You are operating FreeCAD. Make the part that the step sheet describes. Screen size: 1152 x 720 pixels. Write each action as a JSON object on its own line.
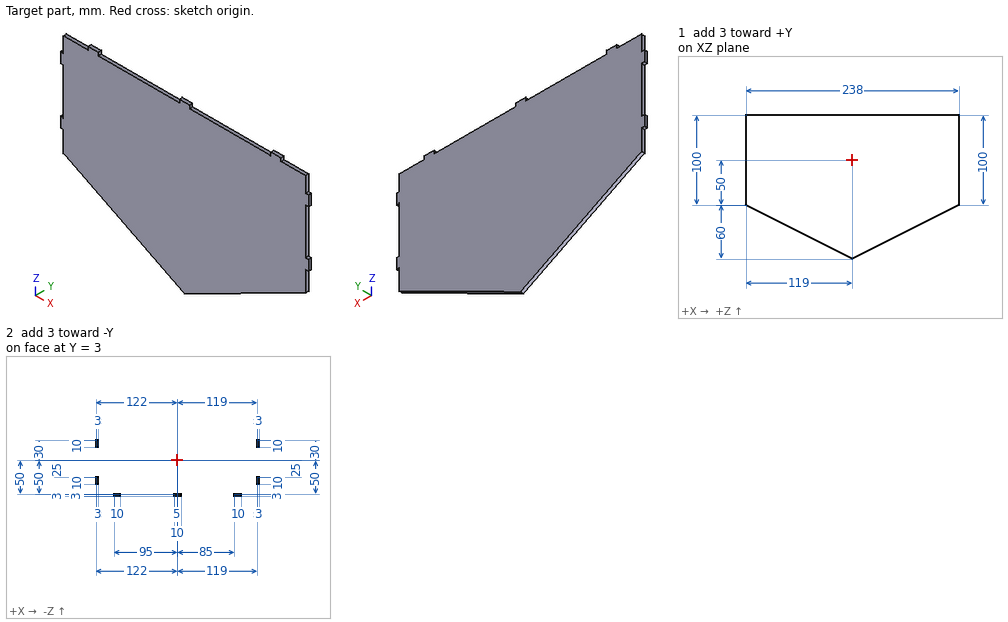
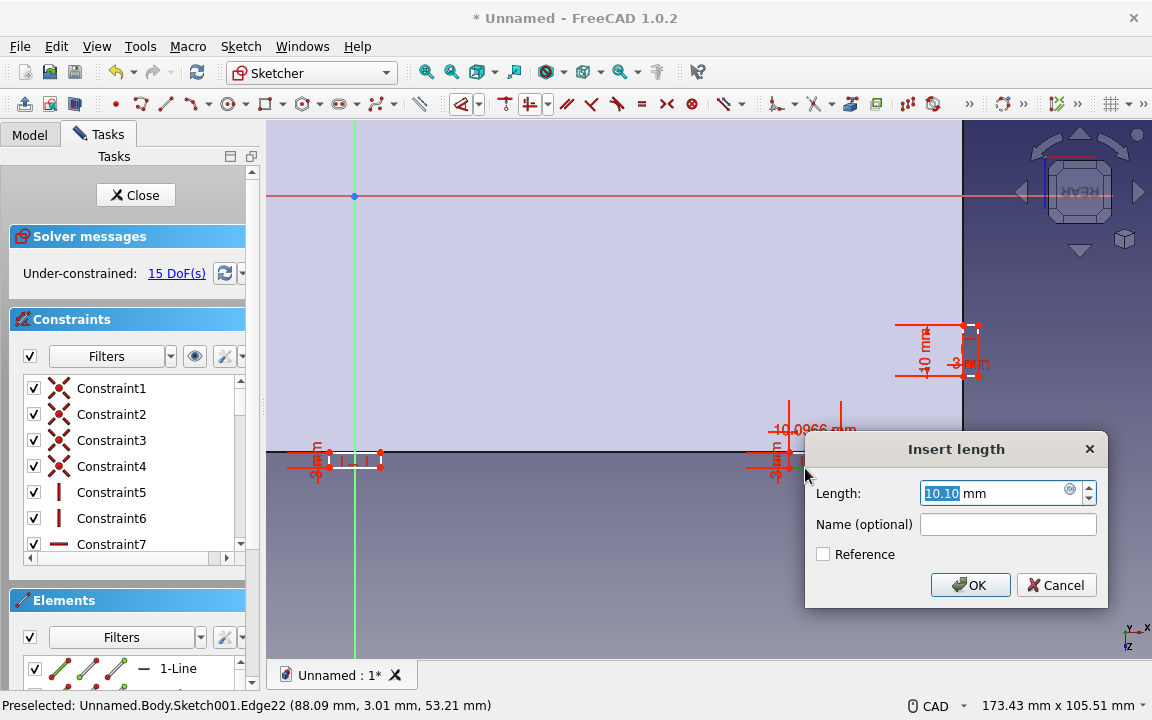
{"action": "type", "text": "10"}
{"action": "key", "text": "Return"}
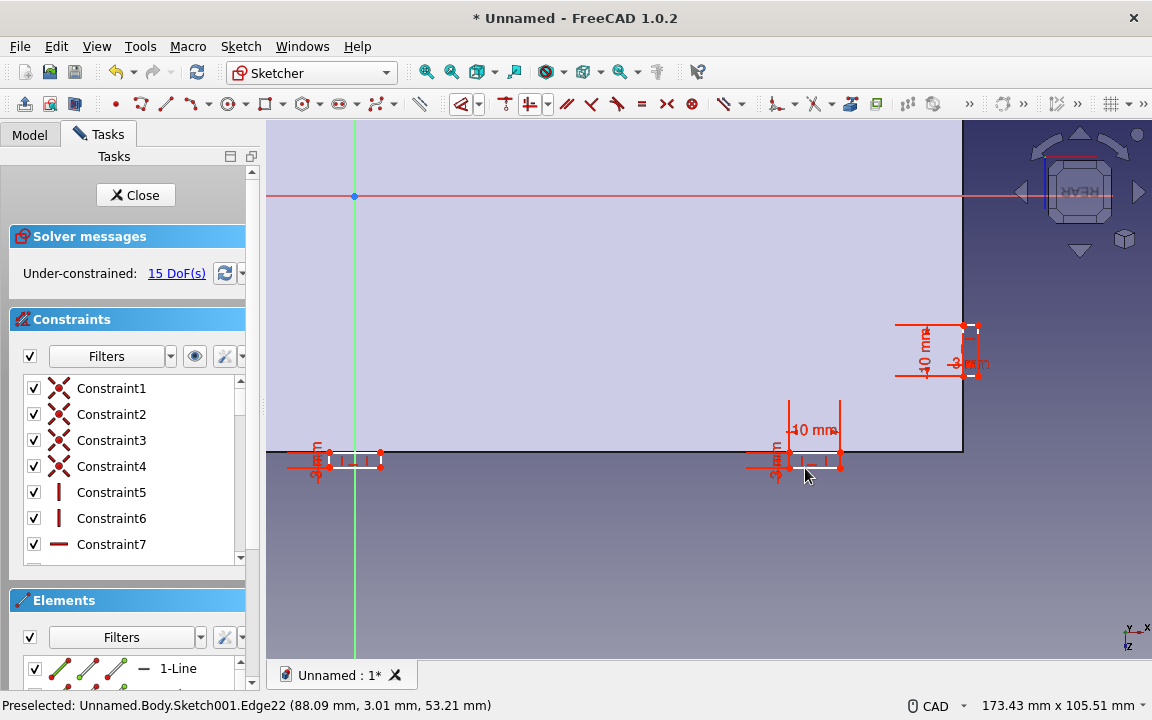
{"action": "scroll", "coordinate": [345, 468], "scroll_direction": "up", "scroll_amount": 2}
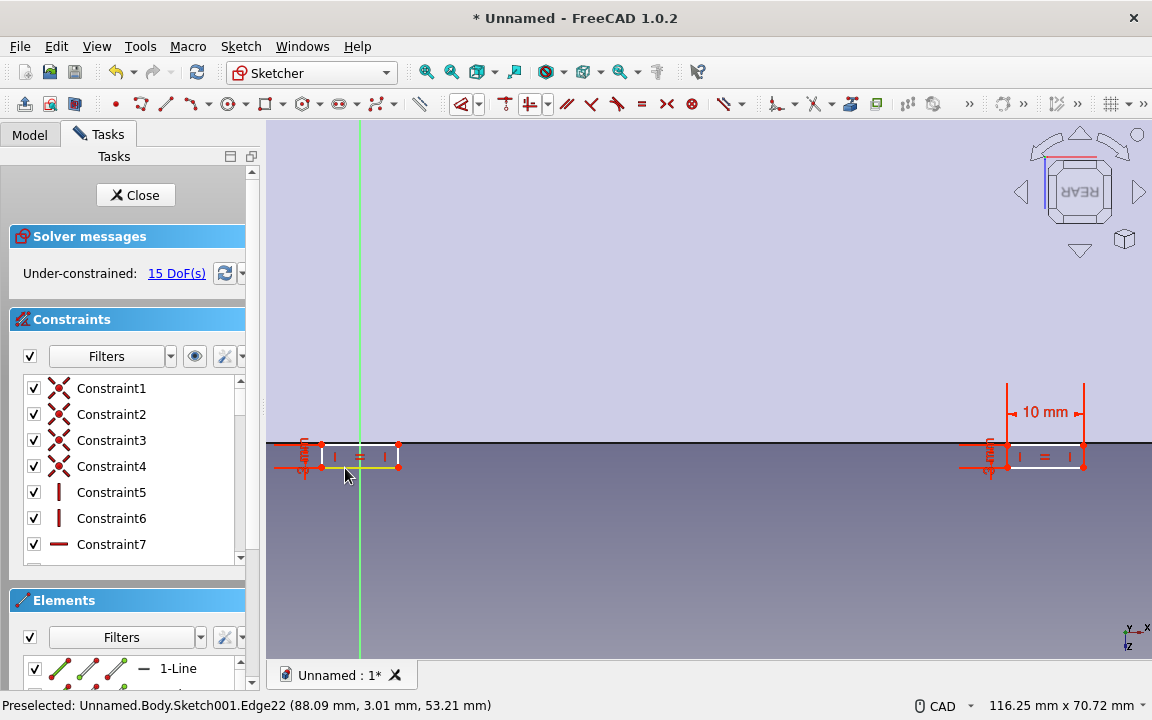
{"action": "left_click", "coordinate": [345, 468]}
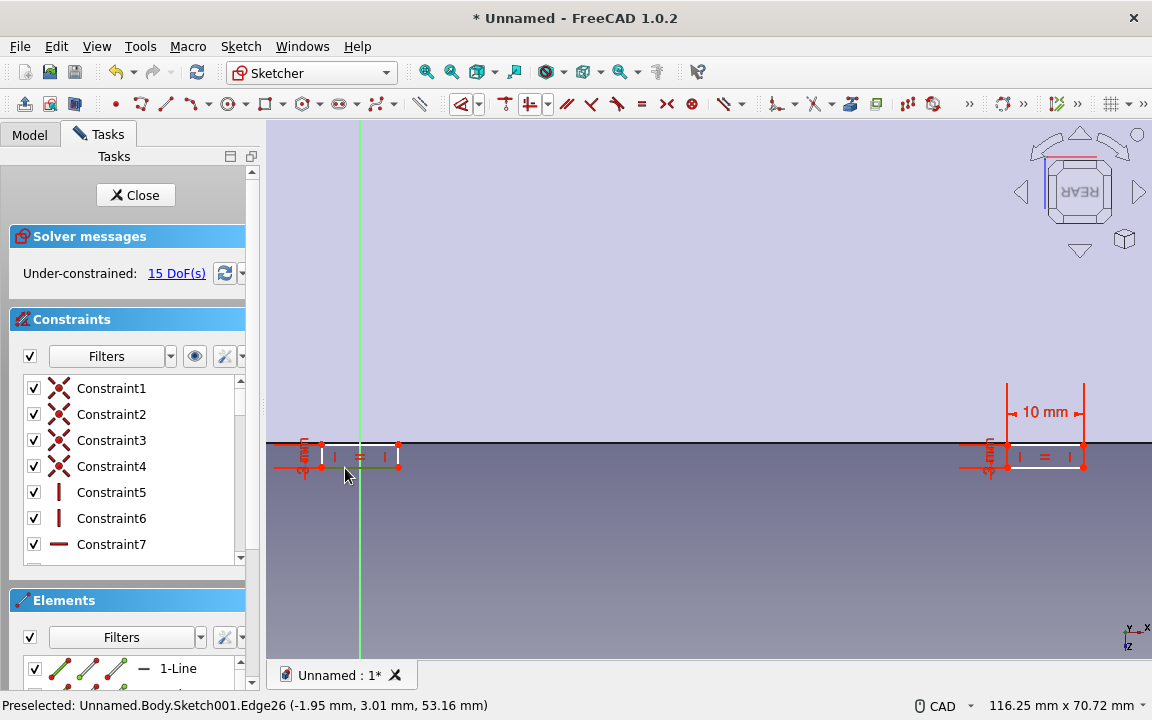
{"action": "key", "text": "l"}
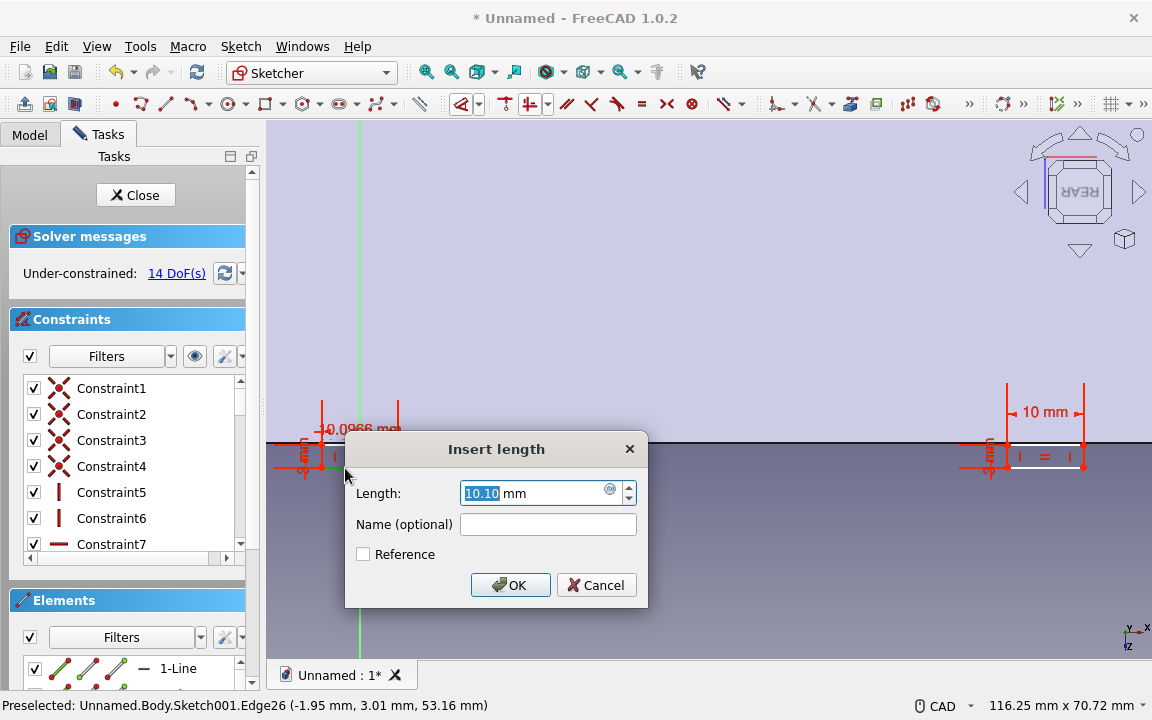
{"action": "type", "text": "10"}
{"action": "key", "text": "Return"}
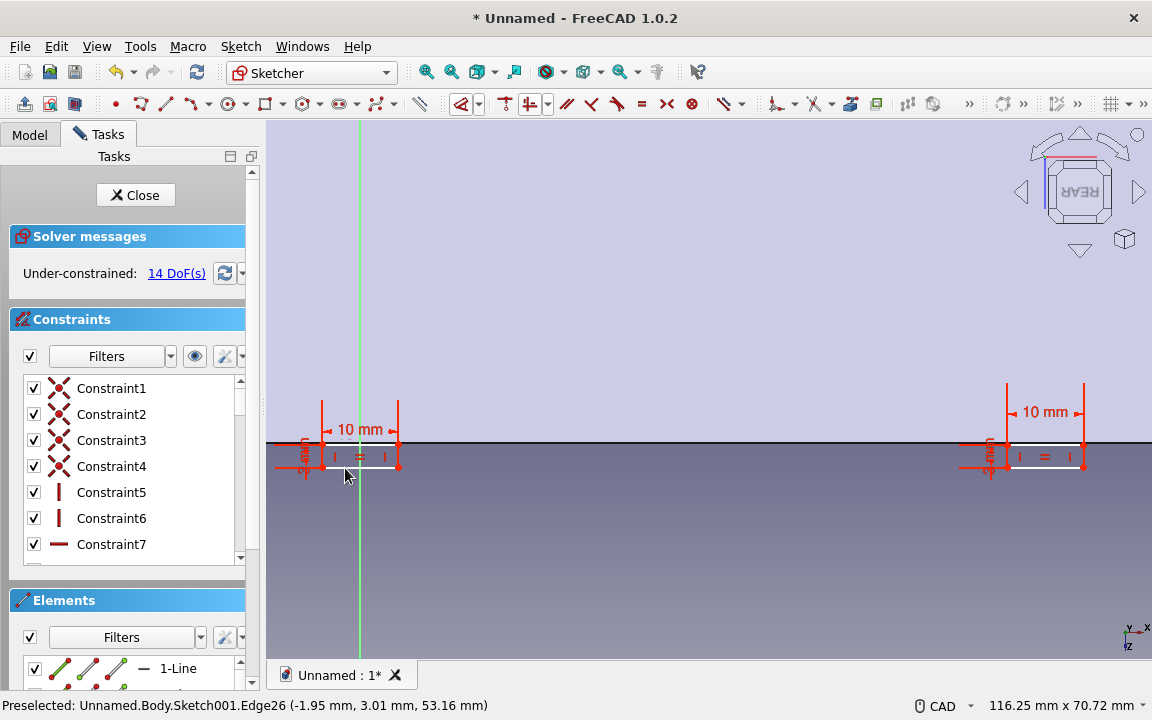
{"action": "left_click", "coordinate": [322, 445]}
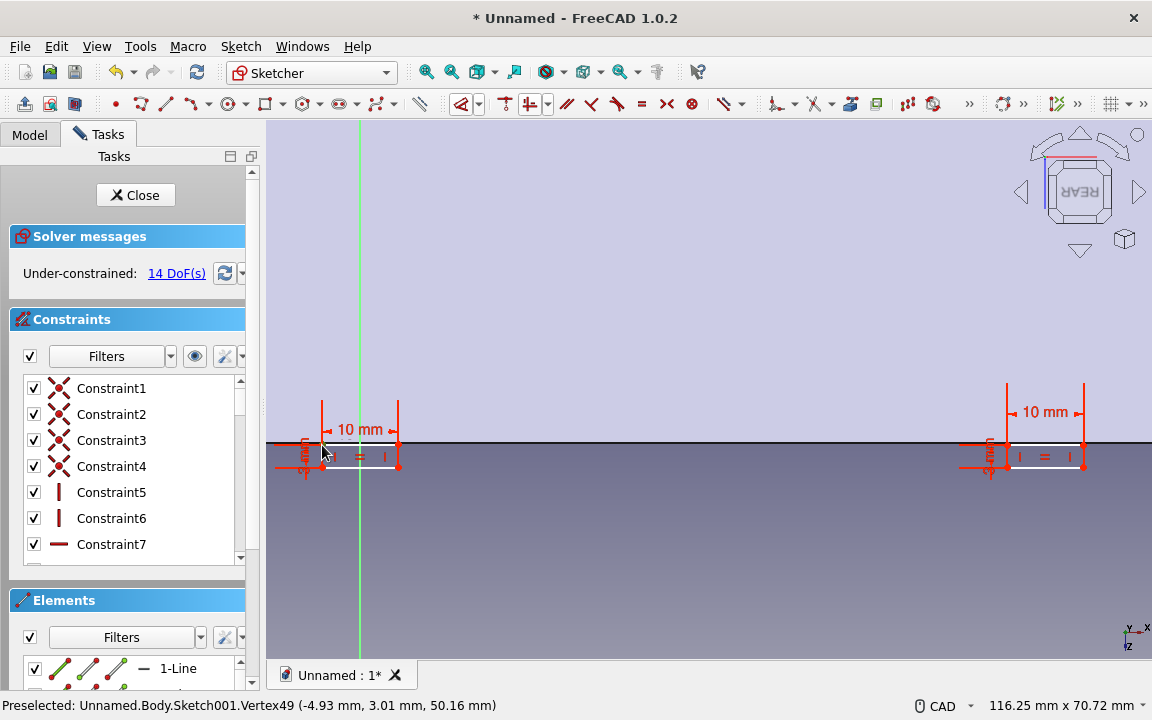
{"action": "key", "text": "l"}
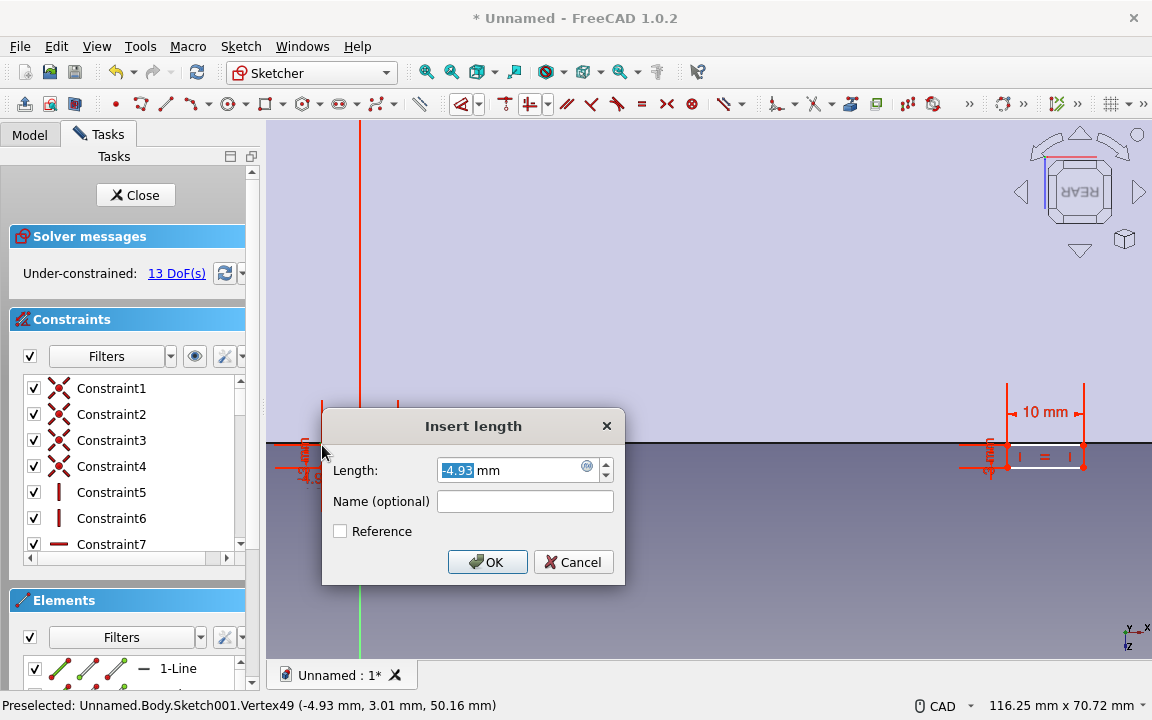
{"action": "type", "text": "-5"}
{"action": "key", "text": "Return"}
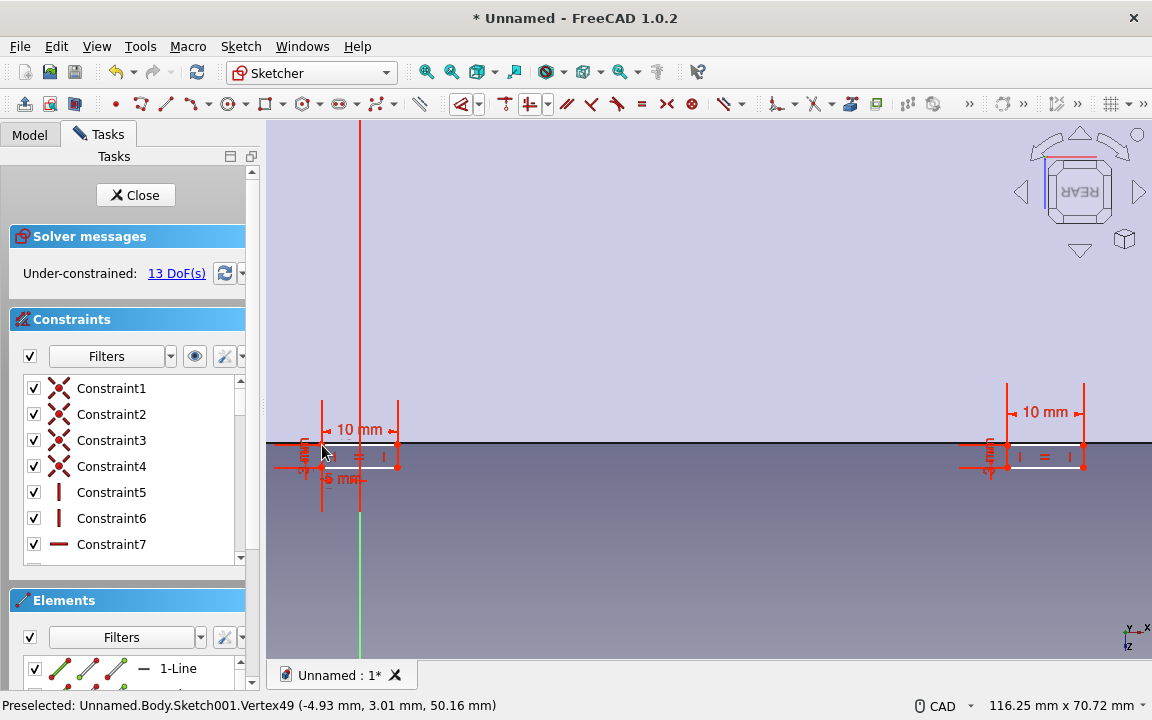
{"action": "scroll", "coordinate": [732, 468], "scroll_direction": "down", "scroll_amount": 7}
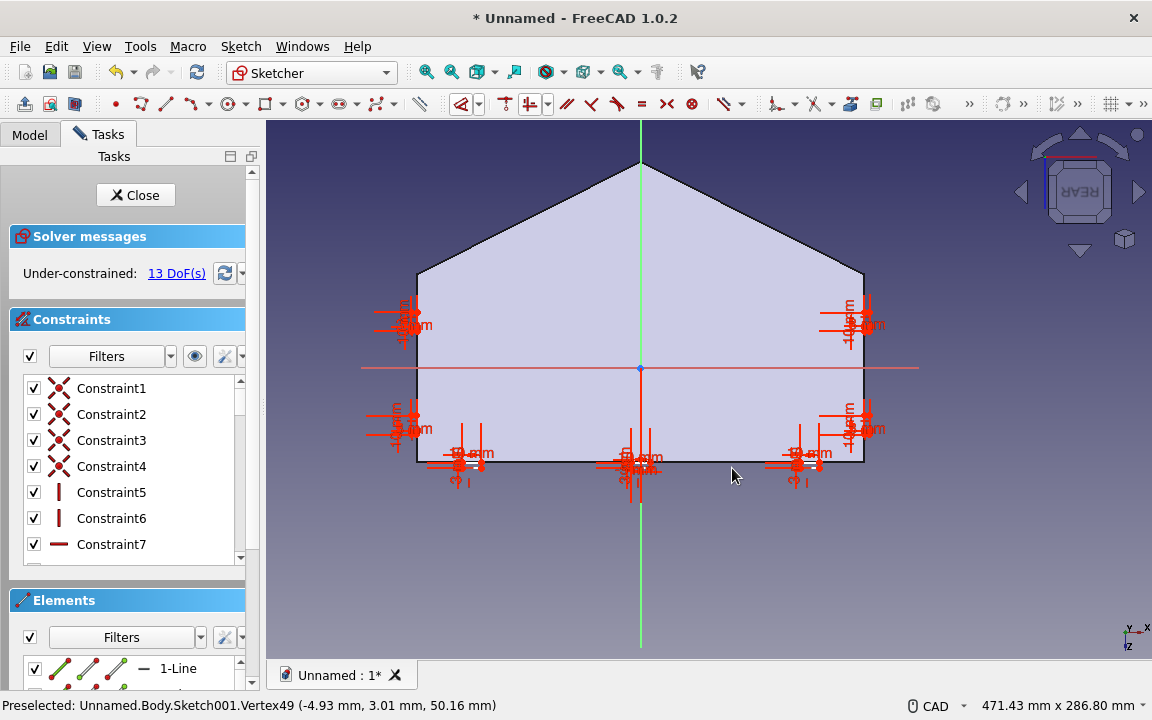
{"action": "scroll", "coordinate": [864, 313], "scroll_direction": "up", "scroll_amount": 4}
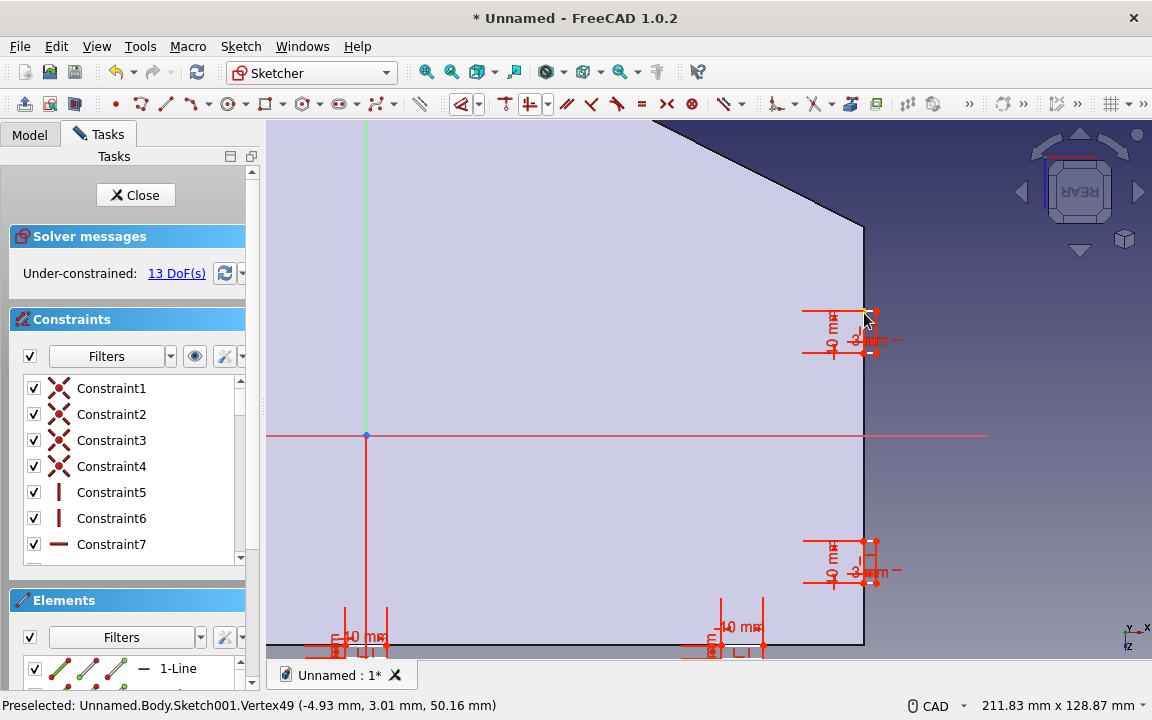
{"action": "left_click", "coordinate": [864, 311]}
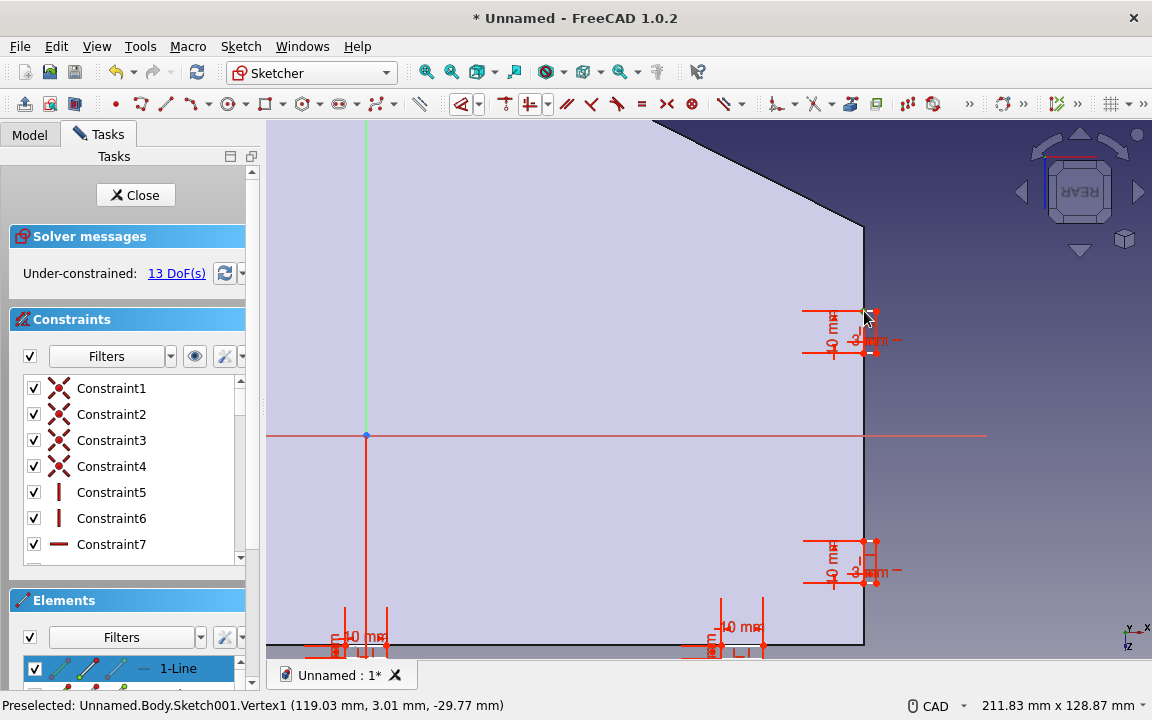
{"action": "key", "text": "i"}